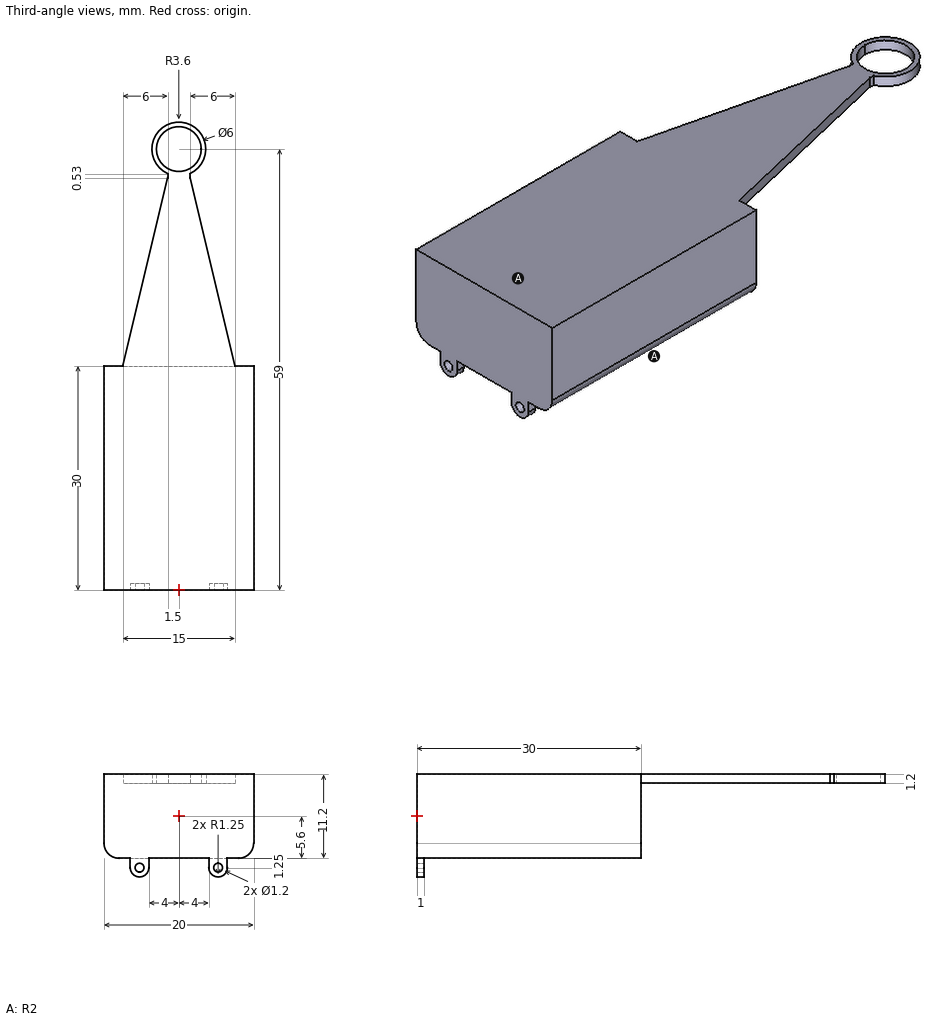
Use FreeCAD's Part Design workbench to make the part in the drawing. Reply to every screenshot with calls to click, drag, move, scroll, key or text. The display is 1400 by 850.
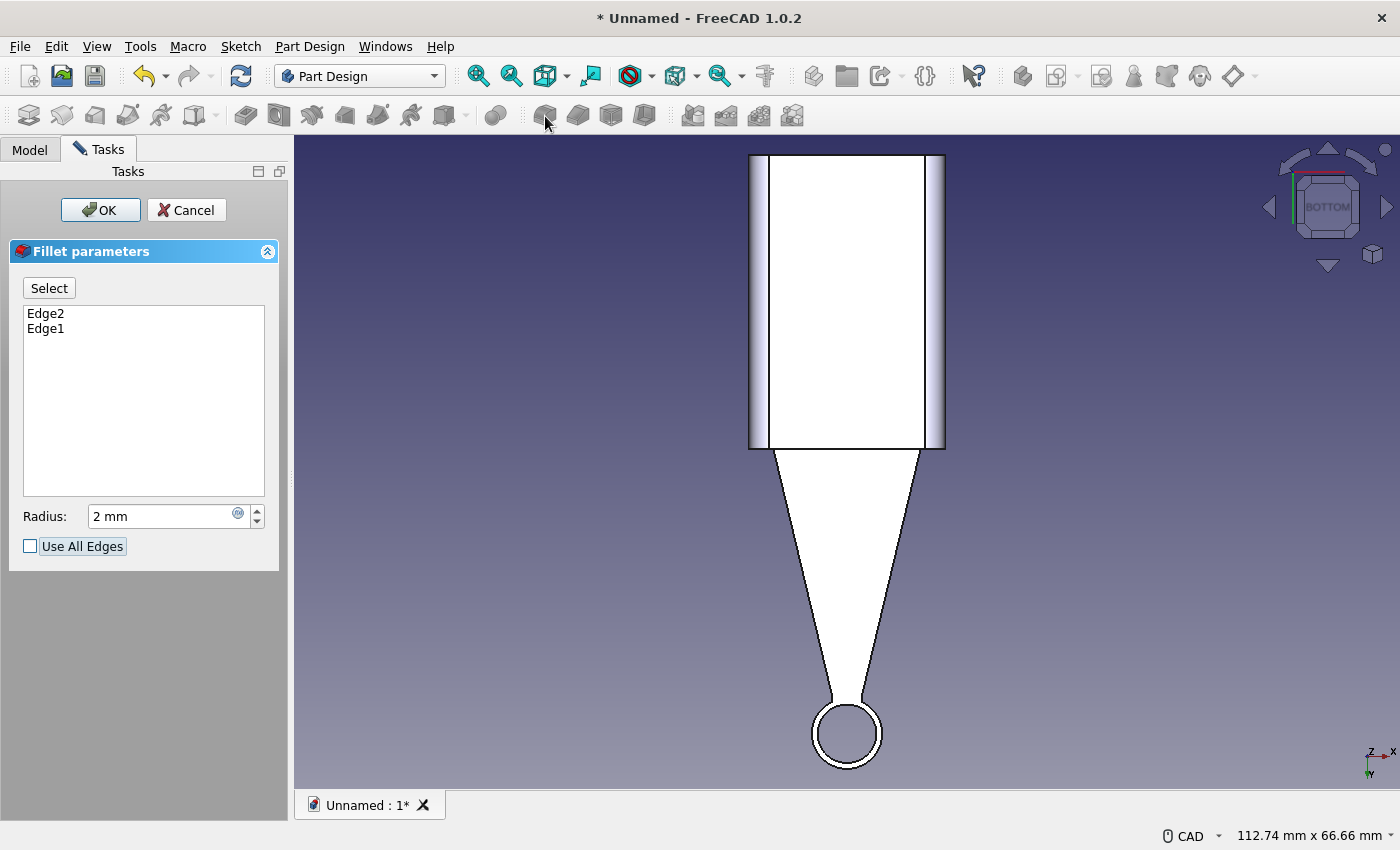
click(101, 210)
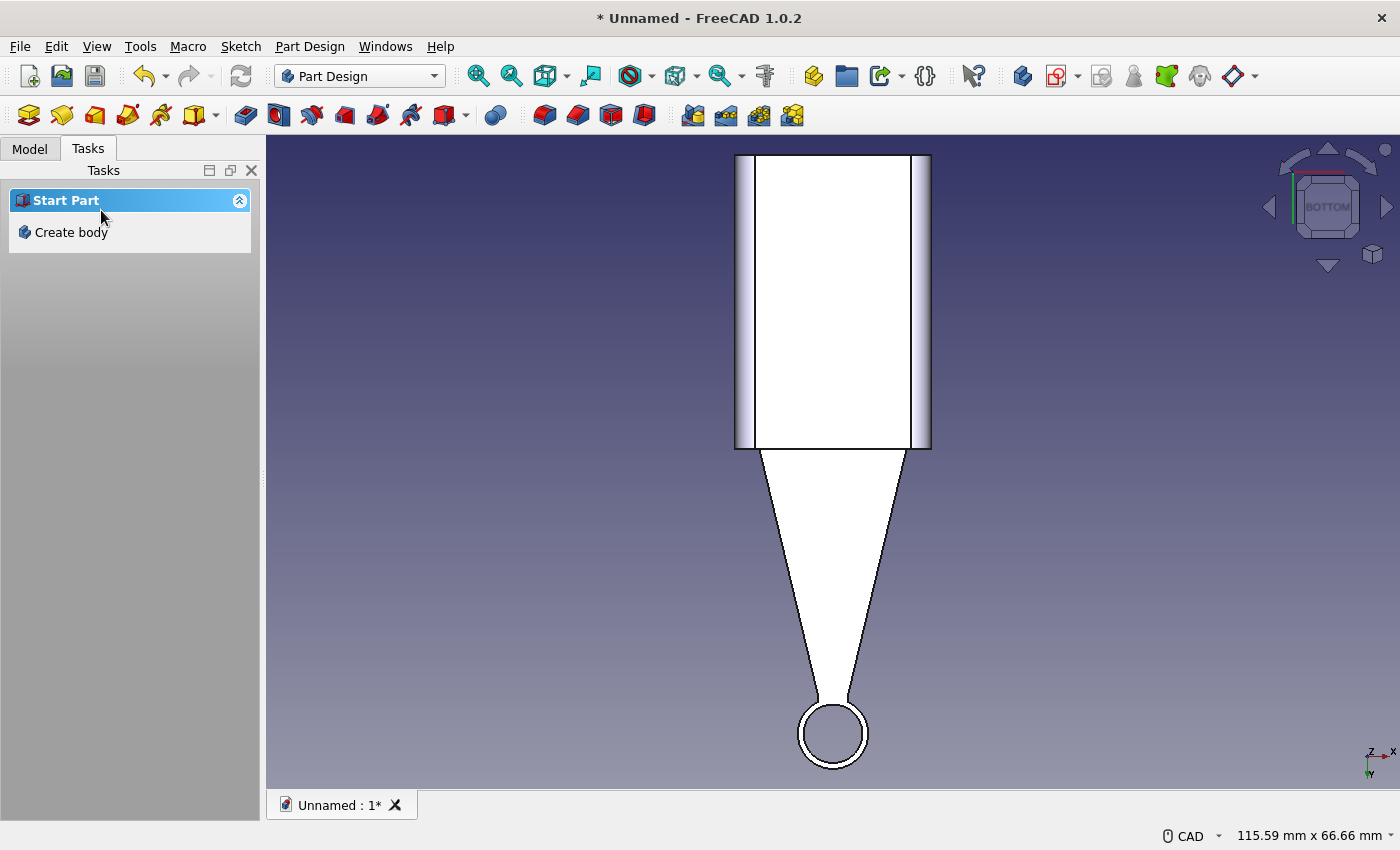
key(0)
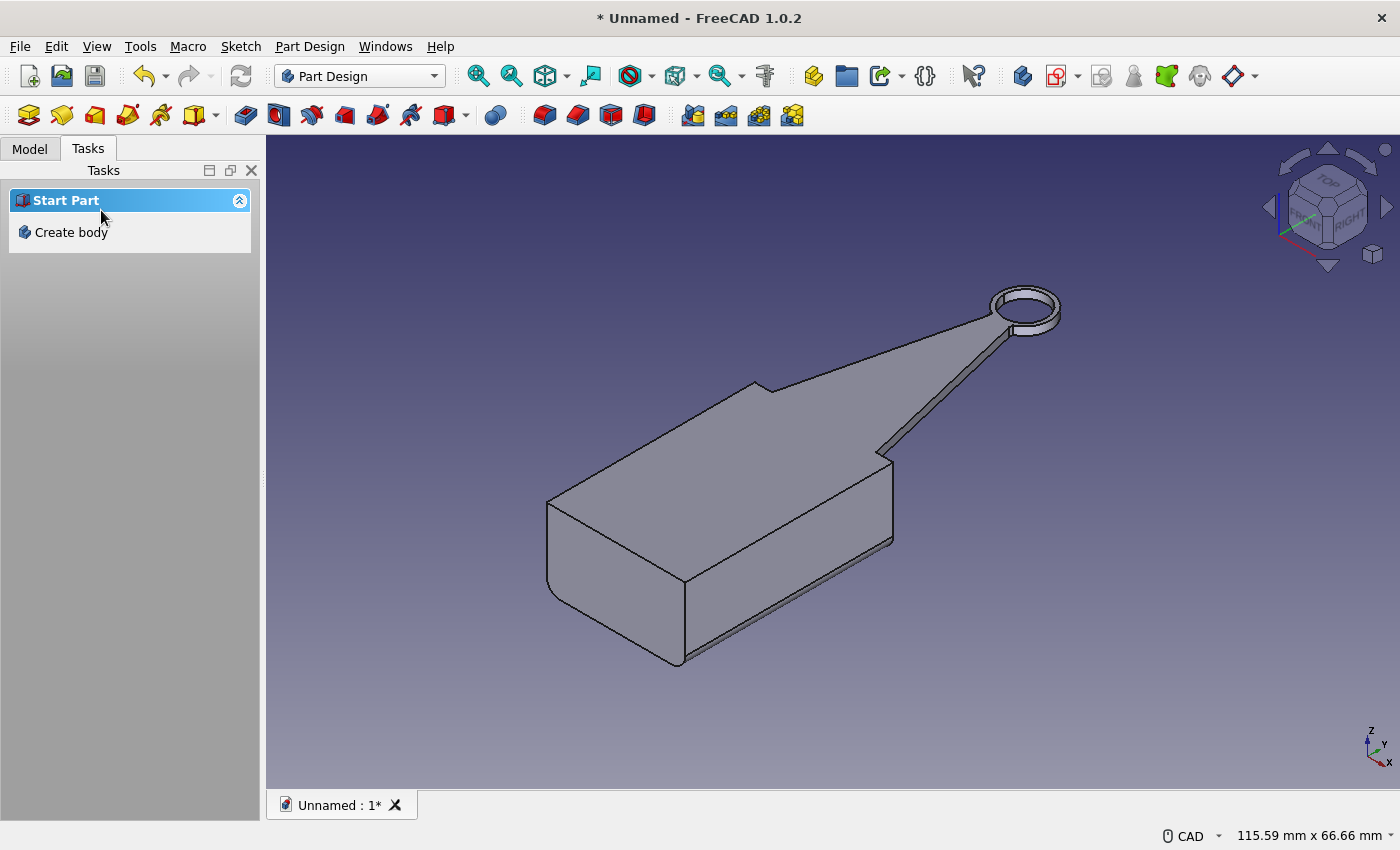
click(636, 598)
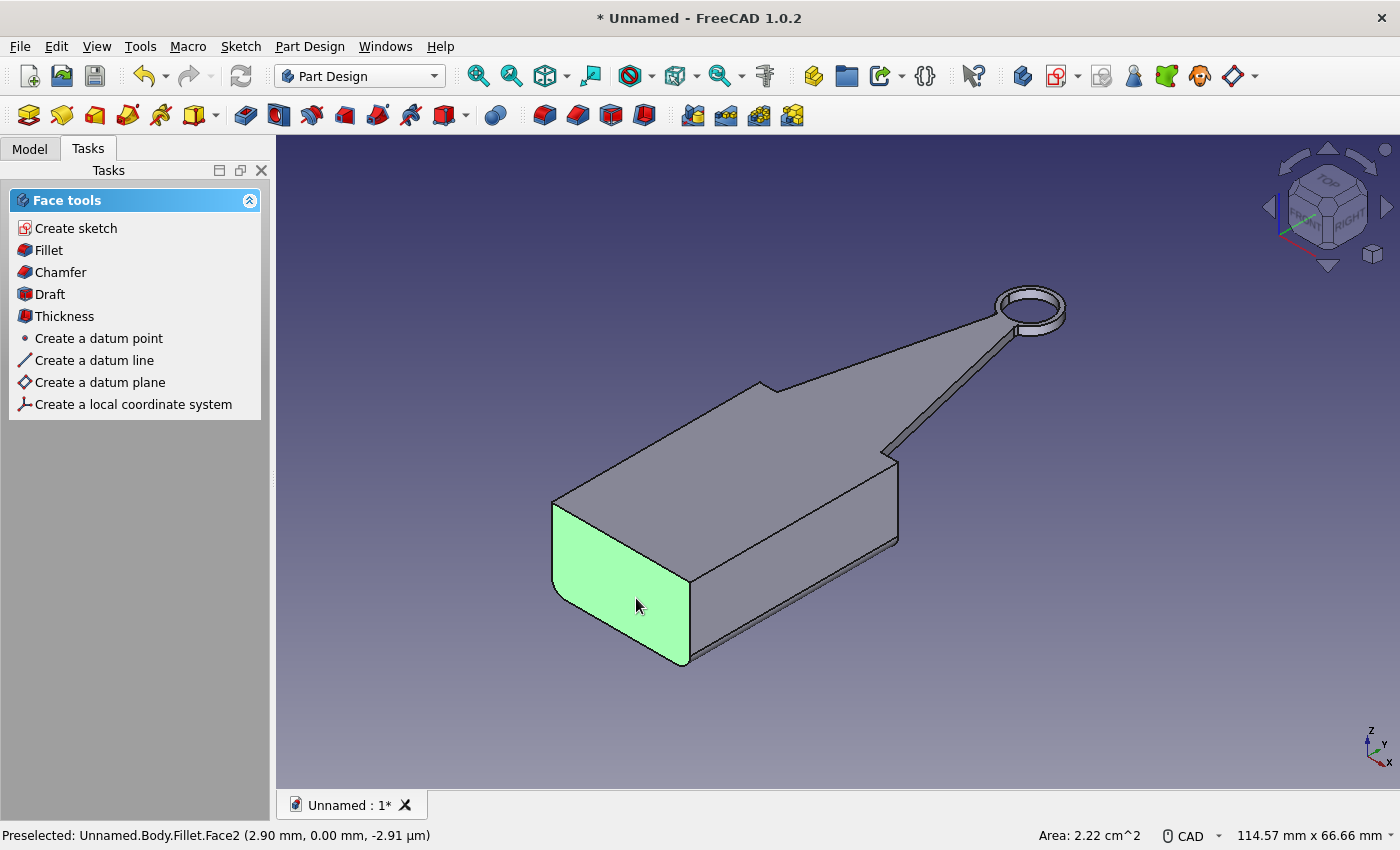
click(1056, 76)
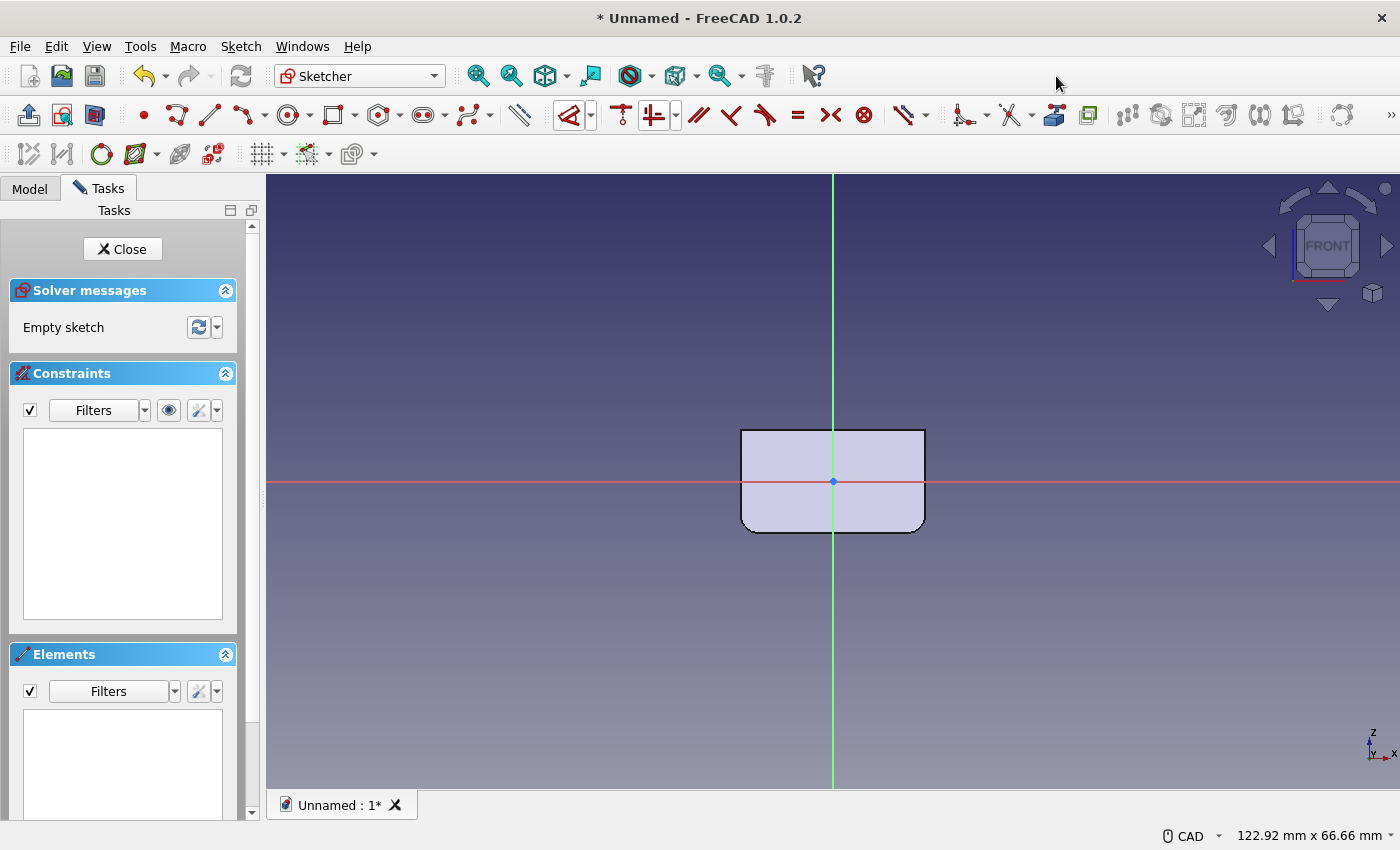
scroll(850, 528, up, 8)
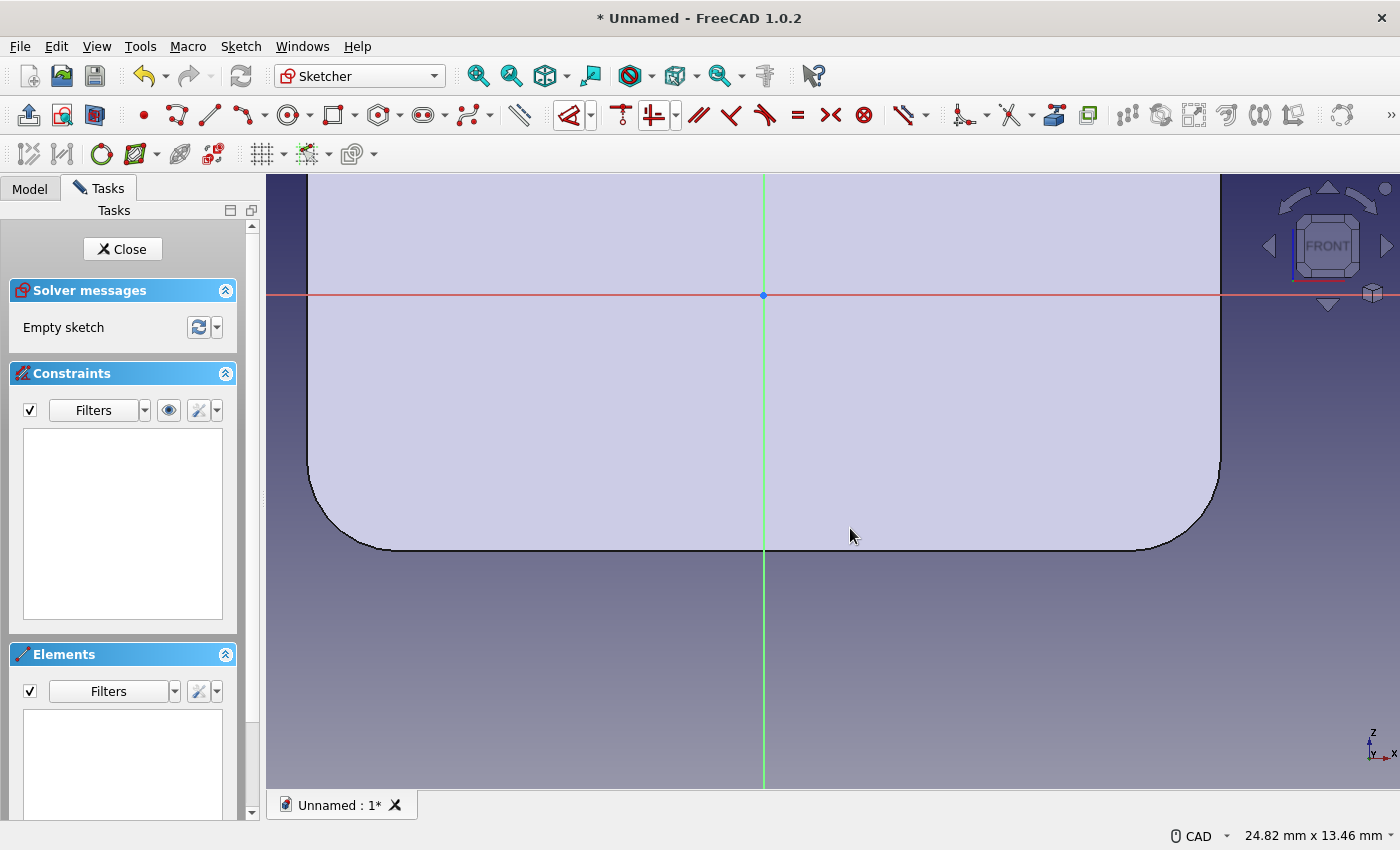
click(177, 116)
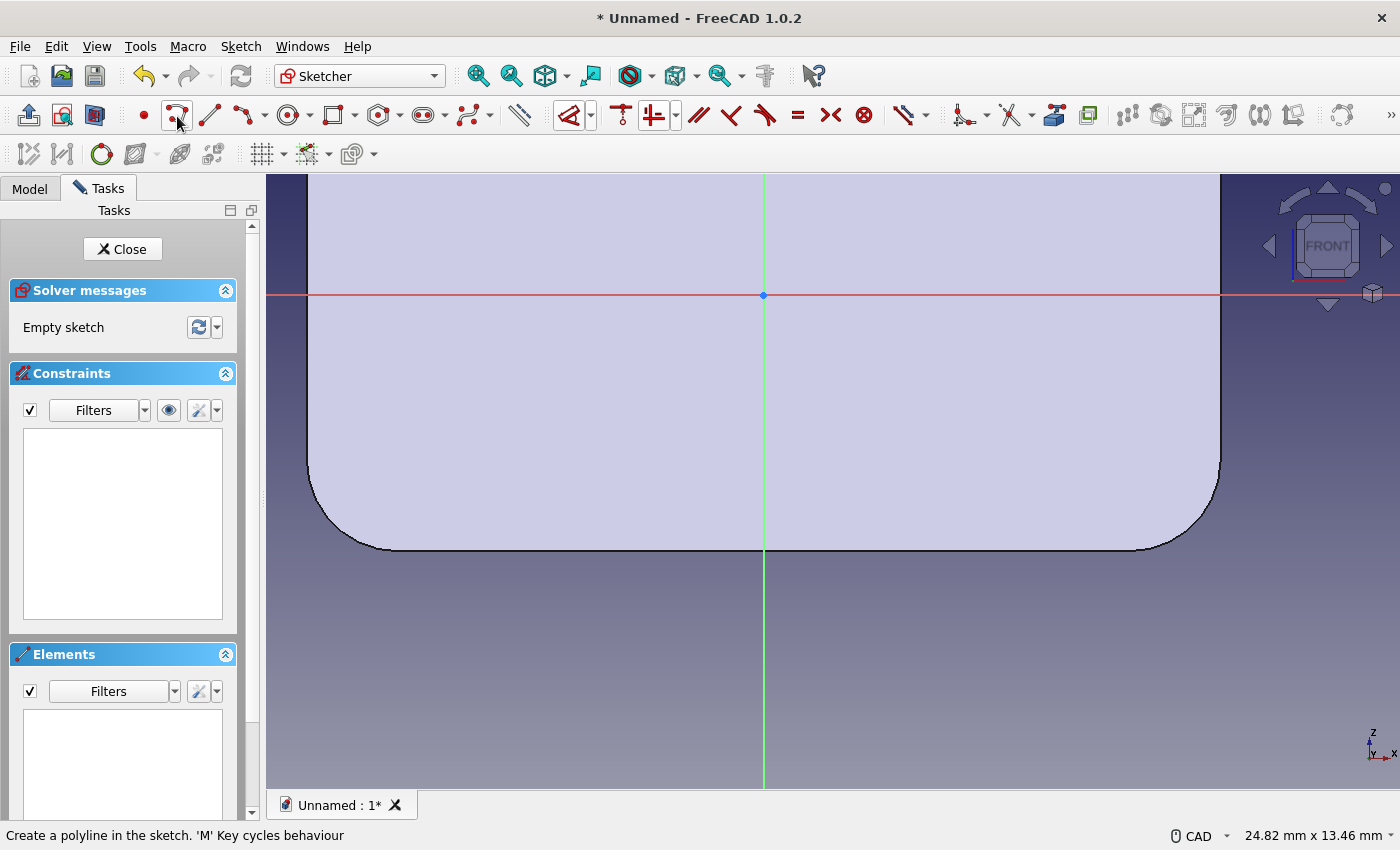
click(1061, 608)
click(1061, 551)
click(947, 551)
click(947, 608)
right_click(947, 608)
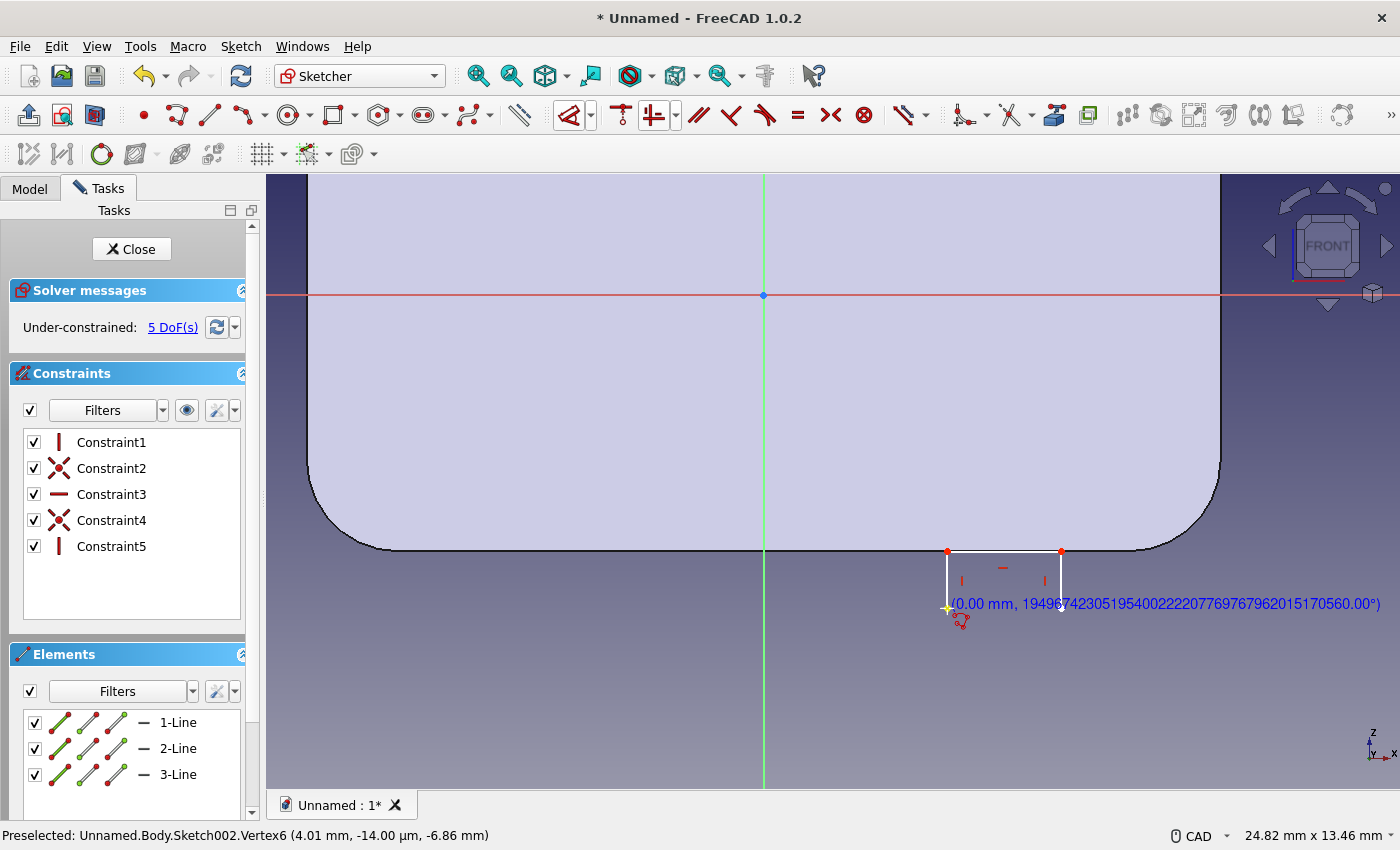
click(242, 116)